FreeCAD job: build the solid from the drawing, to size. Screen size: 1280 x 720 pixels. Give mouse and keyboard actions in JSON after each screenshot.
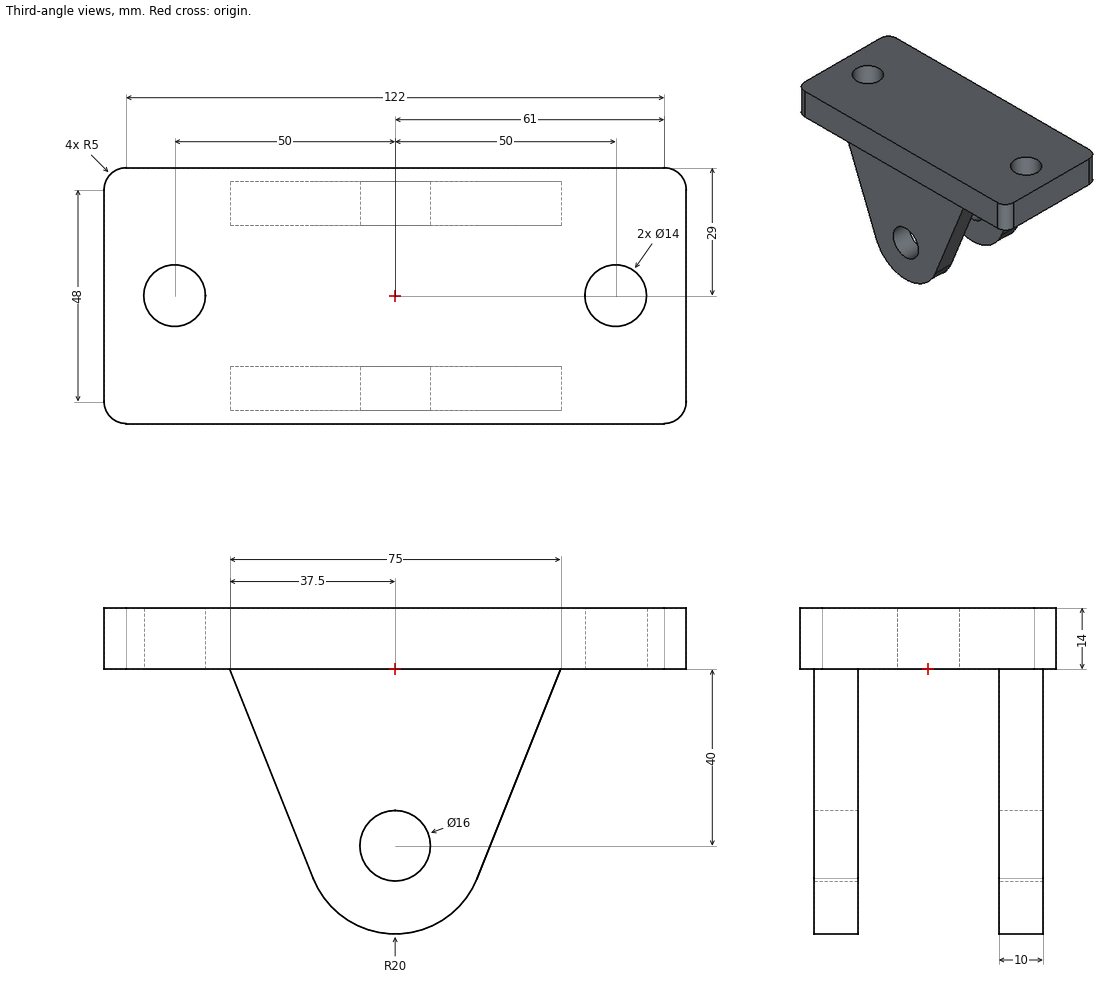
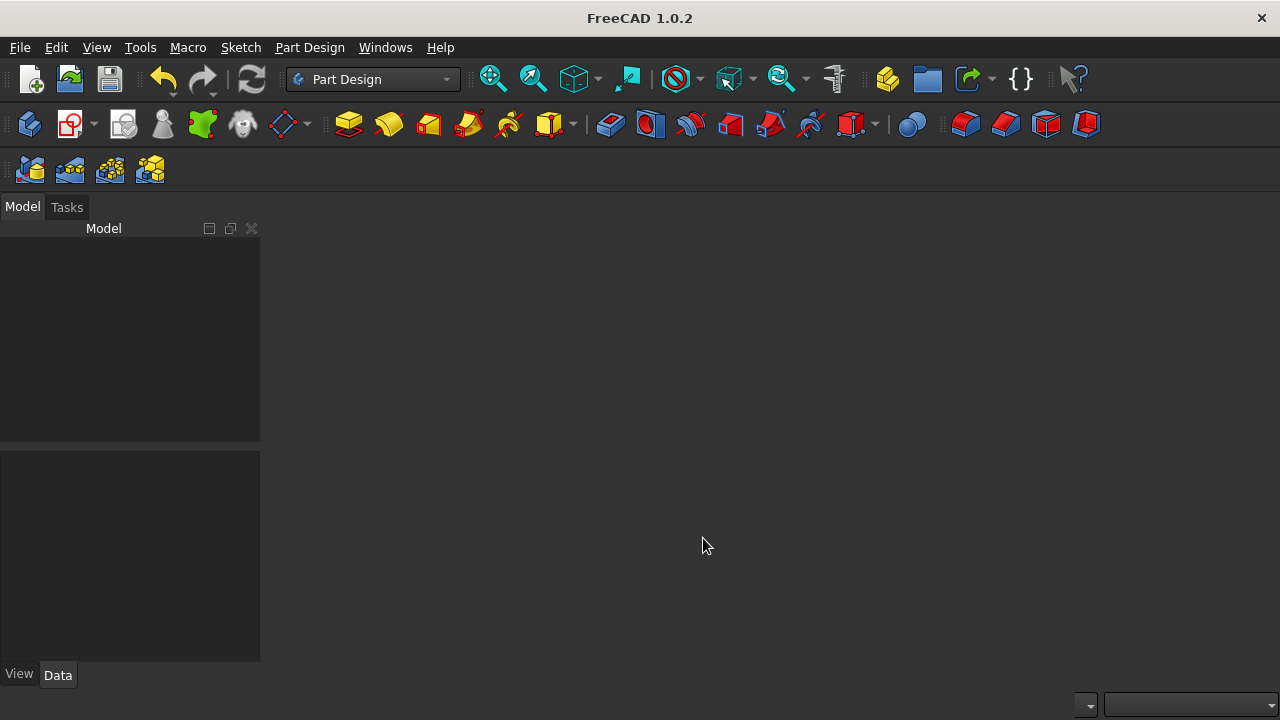
{"action": "left_click", "coordinate": [30, 80]}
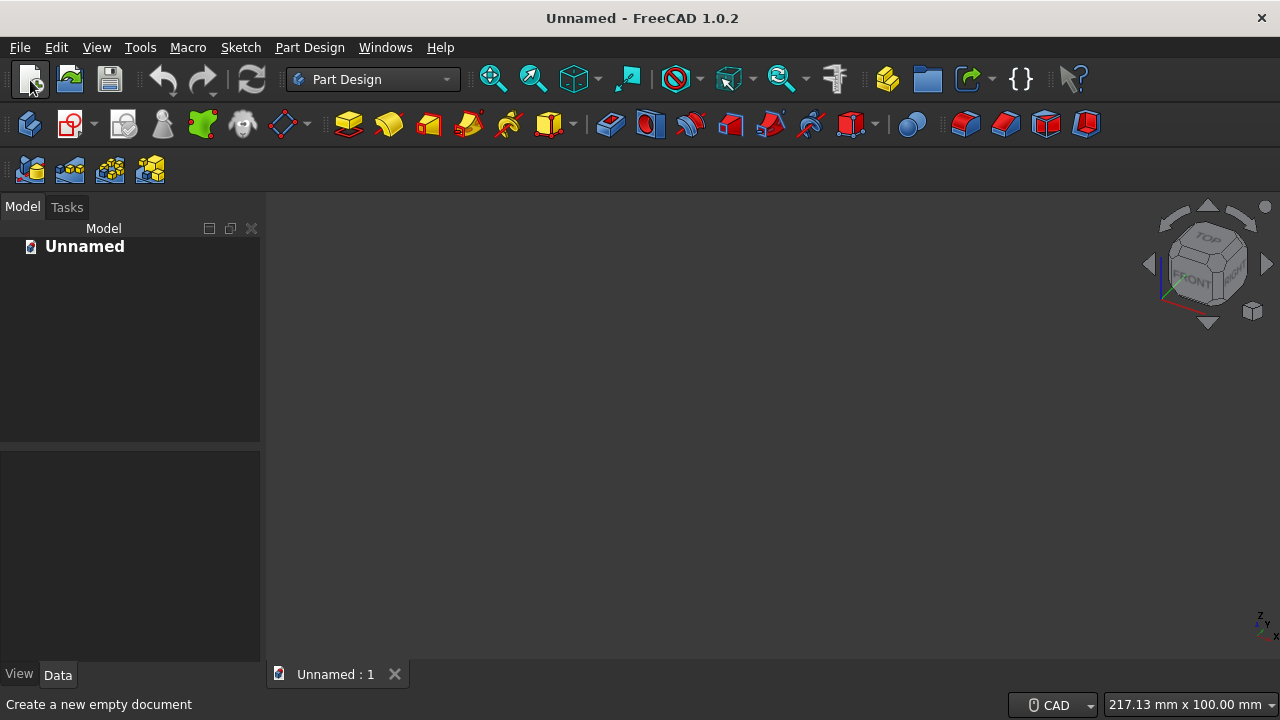
{"action": "left_click", "coordinate": [70, 124]}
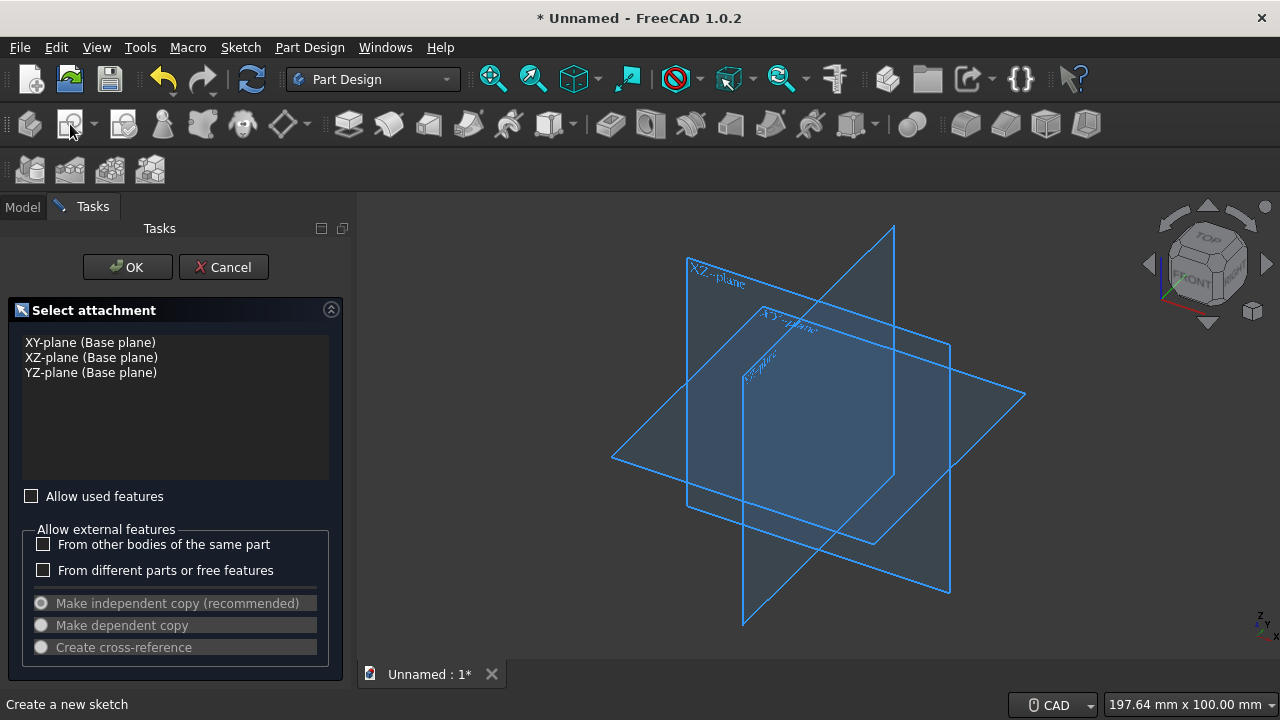
{"action": "left_click", "coordinate": [82, 342]}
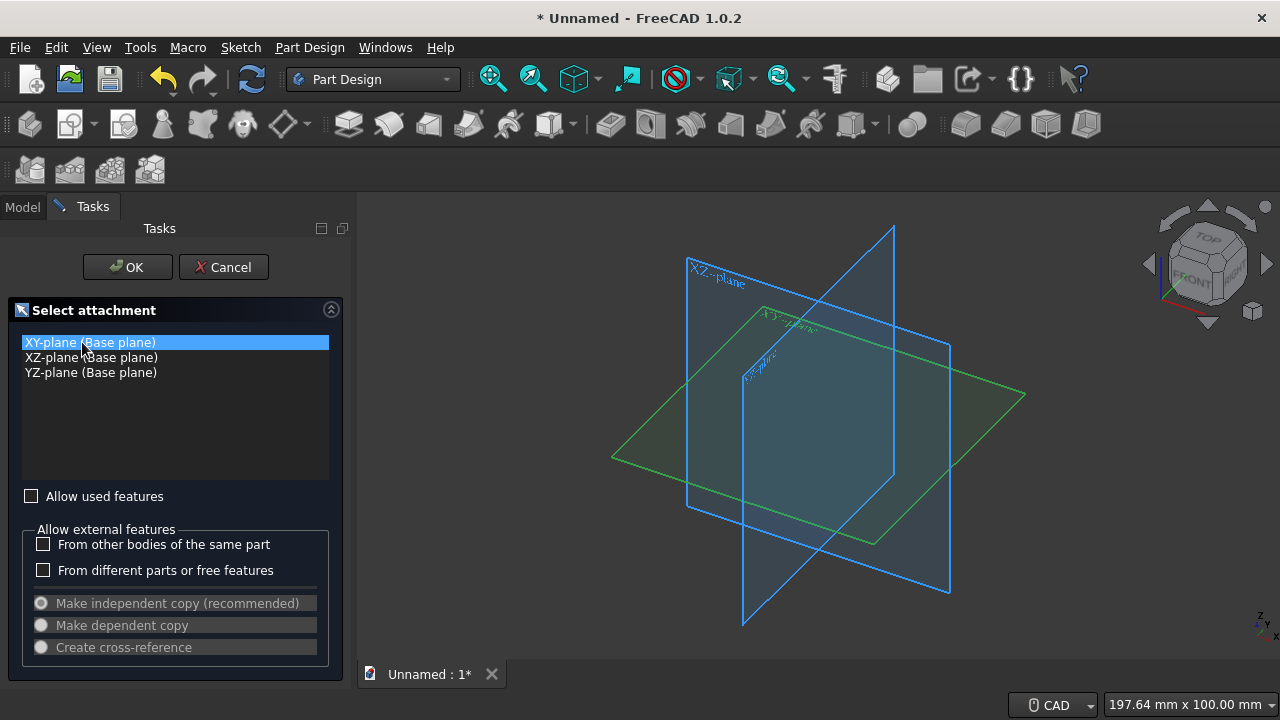
{"action": "left_click", "coordinate": [128, 267]}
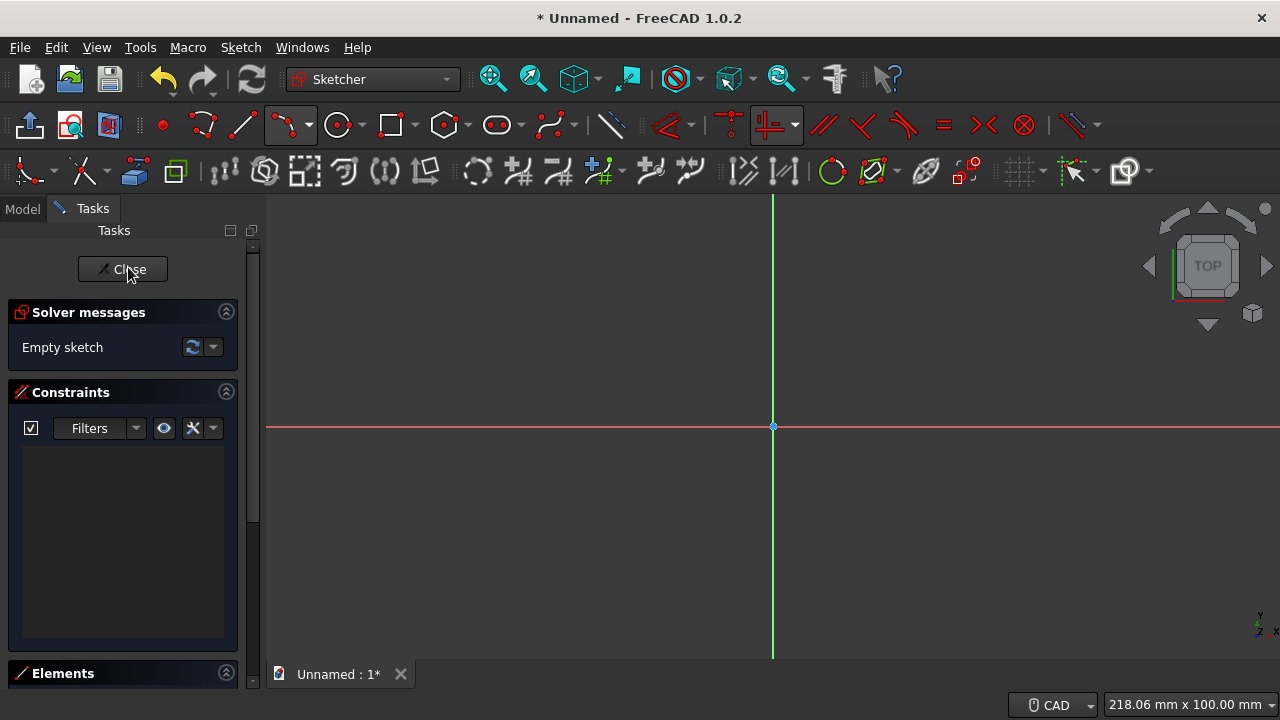
{"action": "left_click", "coordinate": [244, 126]}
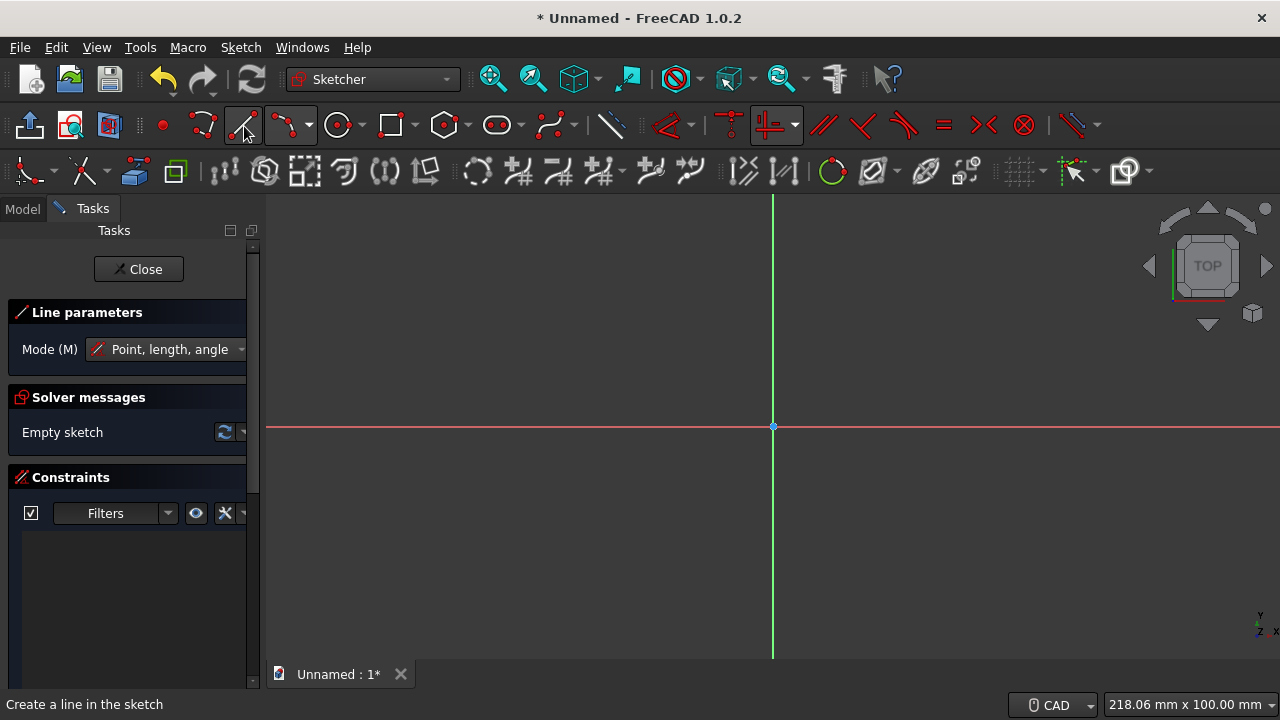
{"action": "left_click", "coordinate": [1057, 292]}
{"action": "left_click", "coordinate": [489, 292]}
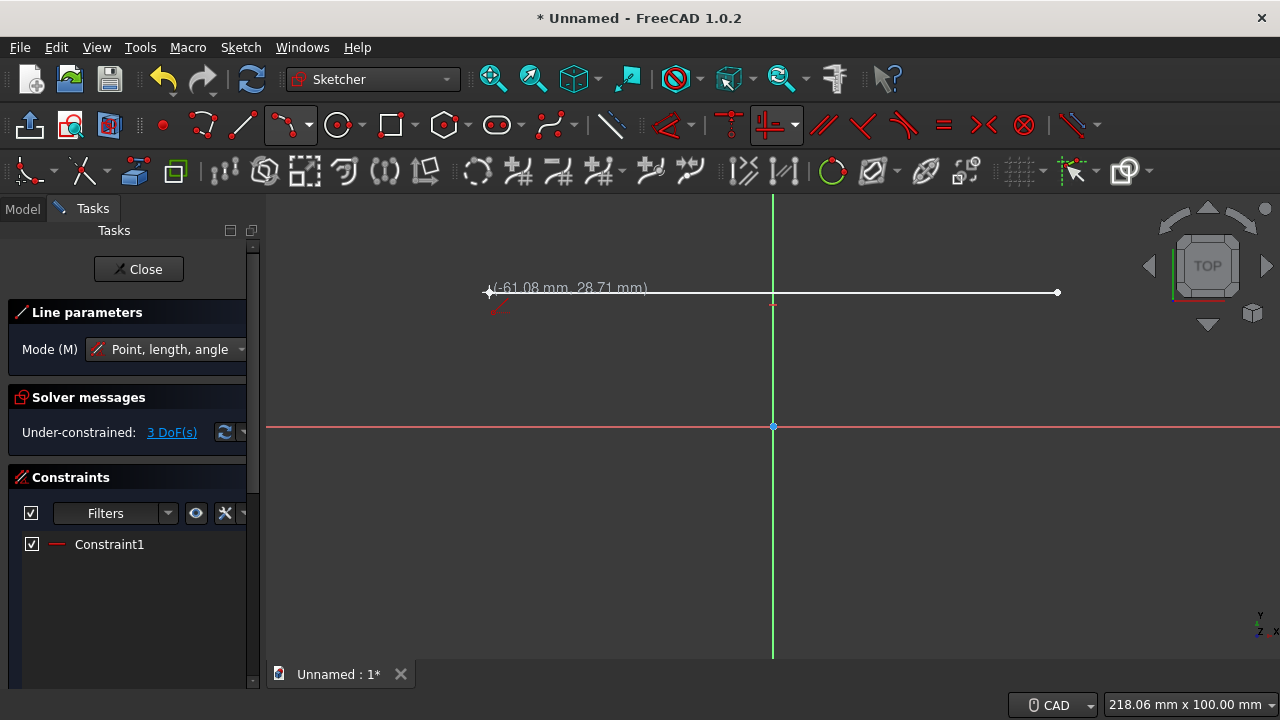
{"action": "left_click", "coordinate": [466, 315]}
{"action": "left_click", "coordinate": [466, 538]}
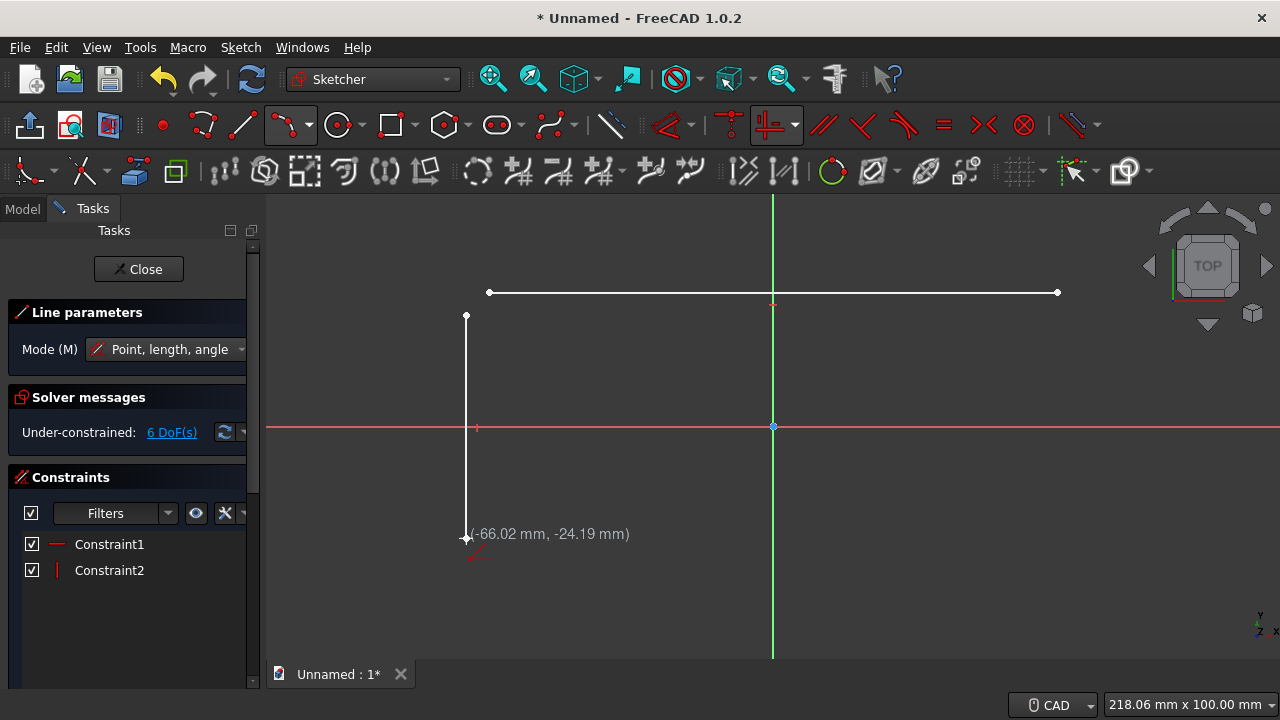
{"action": "left_click", "coordinate": [489, 561]}
{"action": "left_click", "coordinate": [1057, 561]}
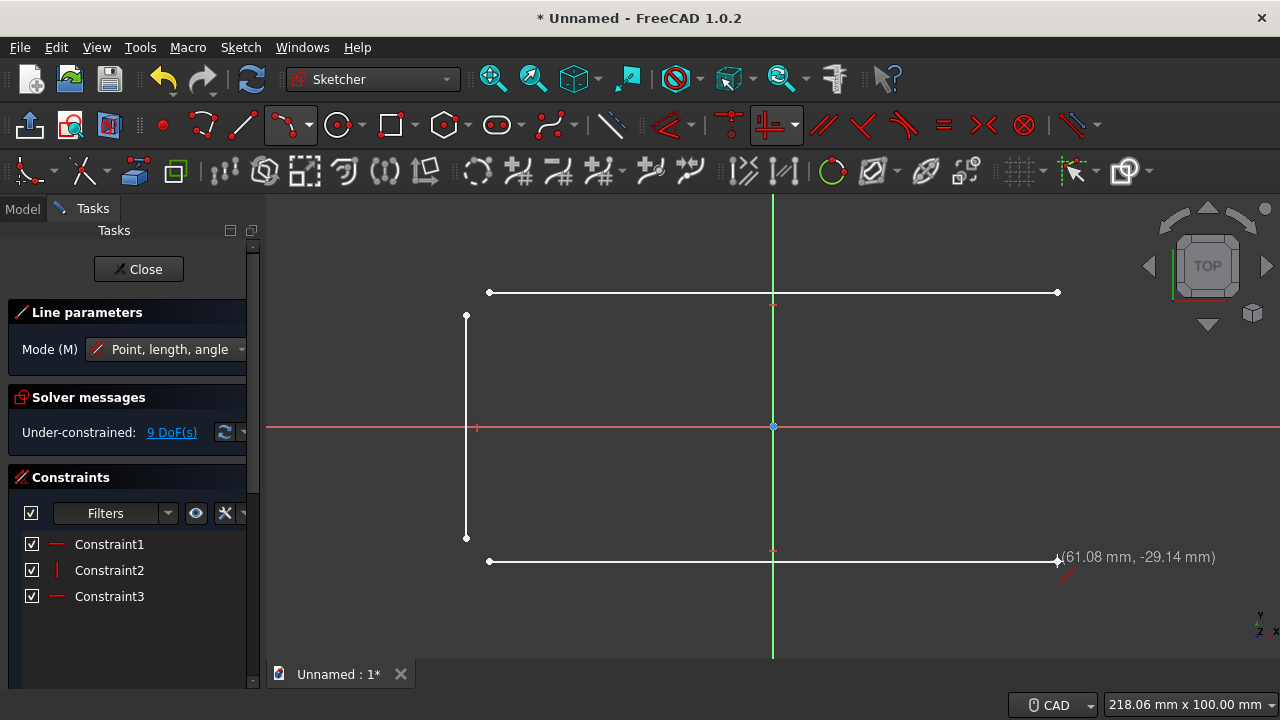
{"action": "left_click", "coordinate": [1080, 538]}
{"action": "left_click", "coordinate": [1080, 315]}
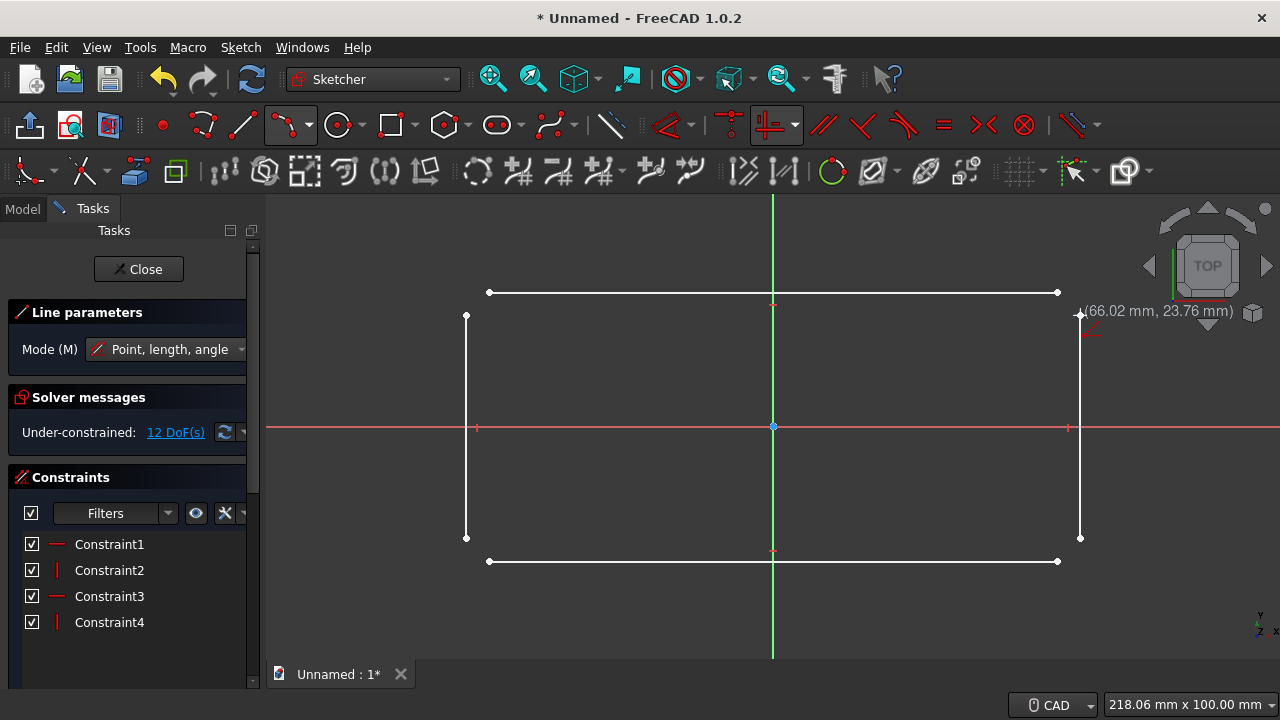
{"action": "left_click", "coordinate": [284, 126]}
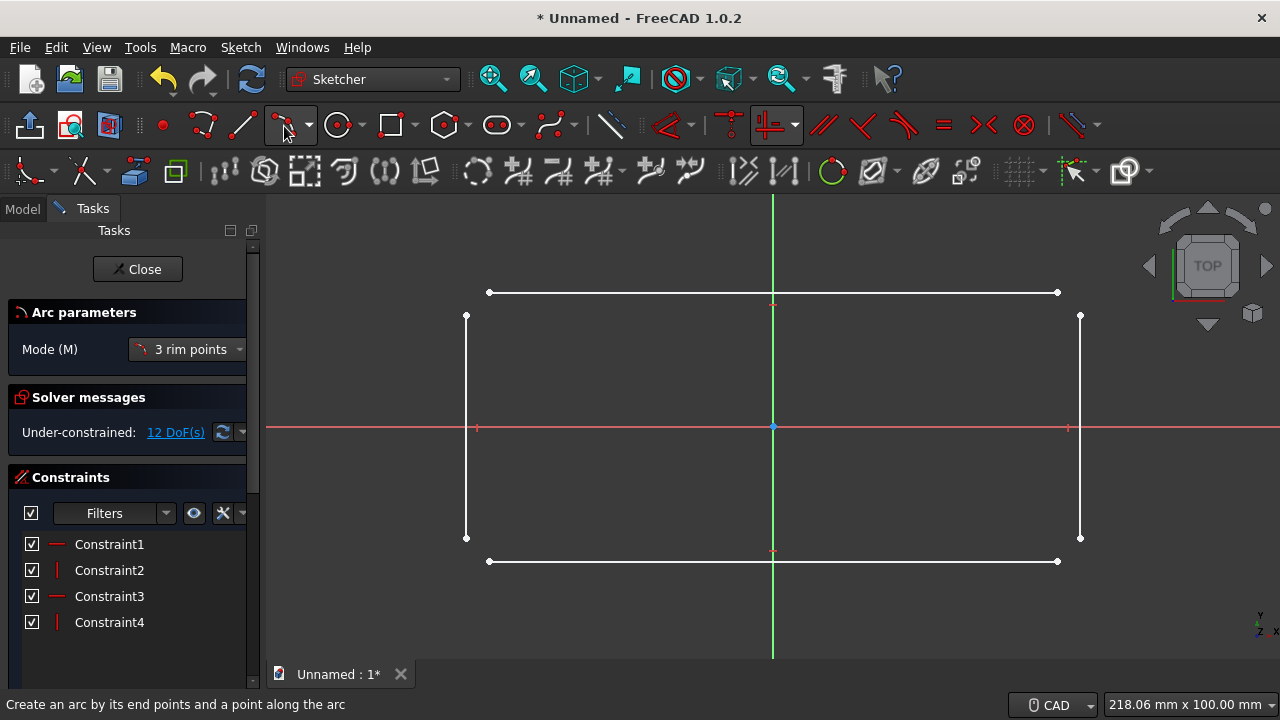
{"action": "left_click", "coordinate": [489, 293]}
{"action": "left_click", "coordinate": [466, 316]}